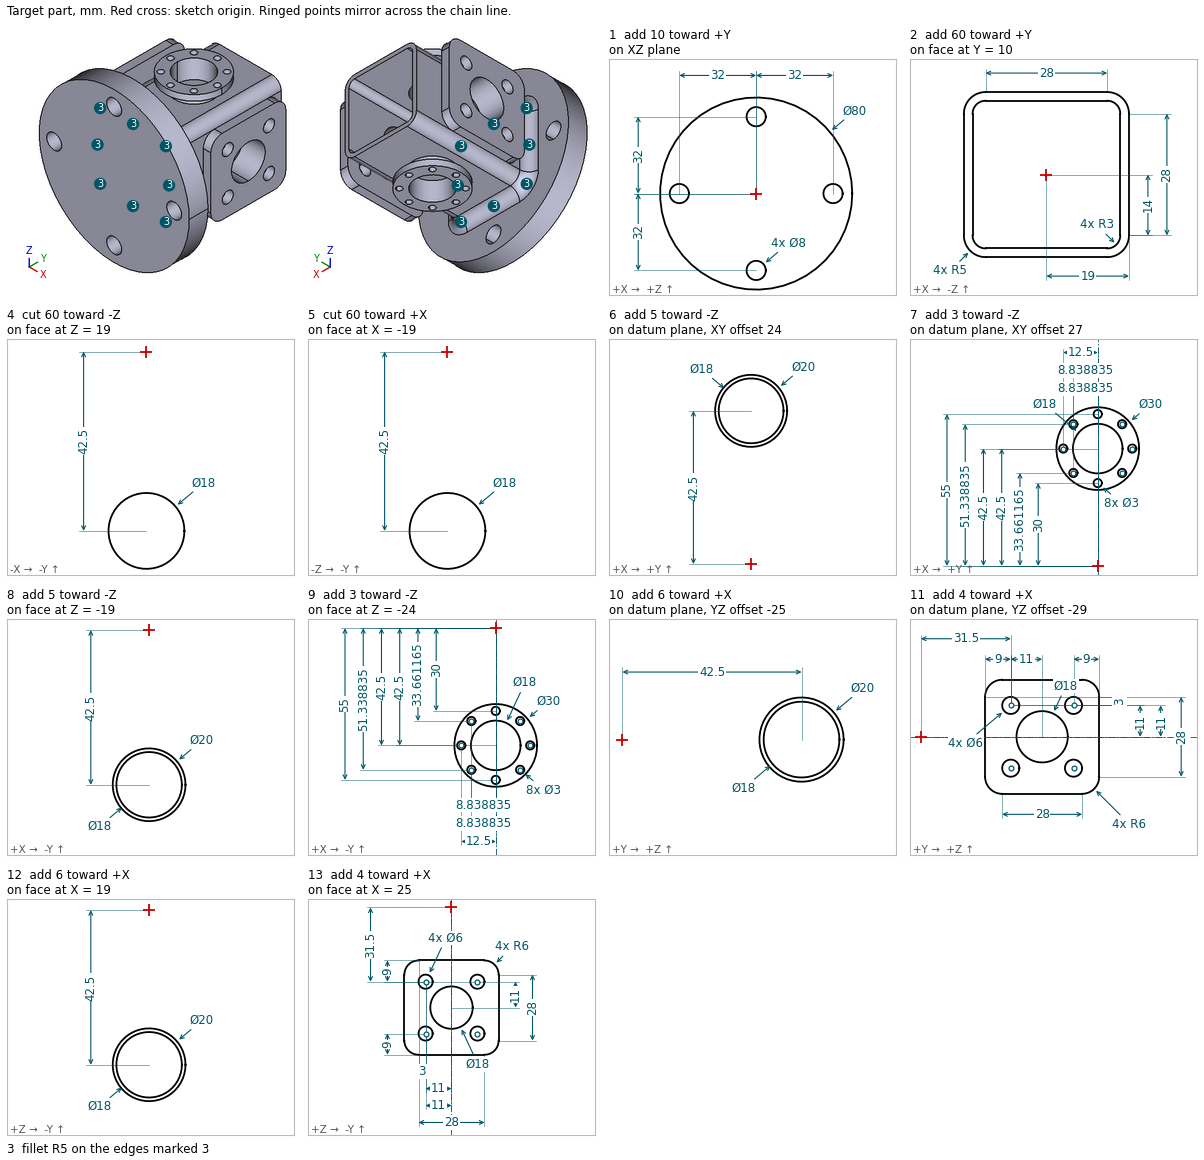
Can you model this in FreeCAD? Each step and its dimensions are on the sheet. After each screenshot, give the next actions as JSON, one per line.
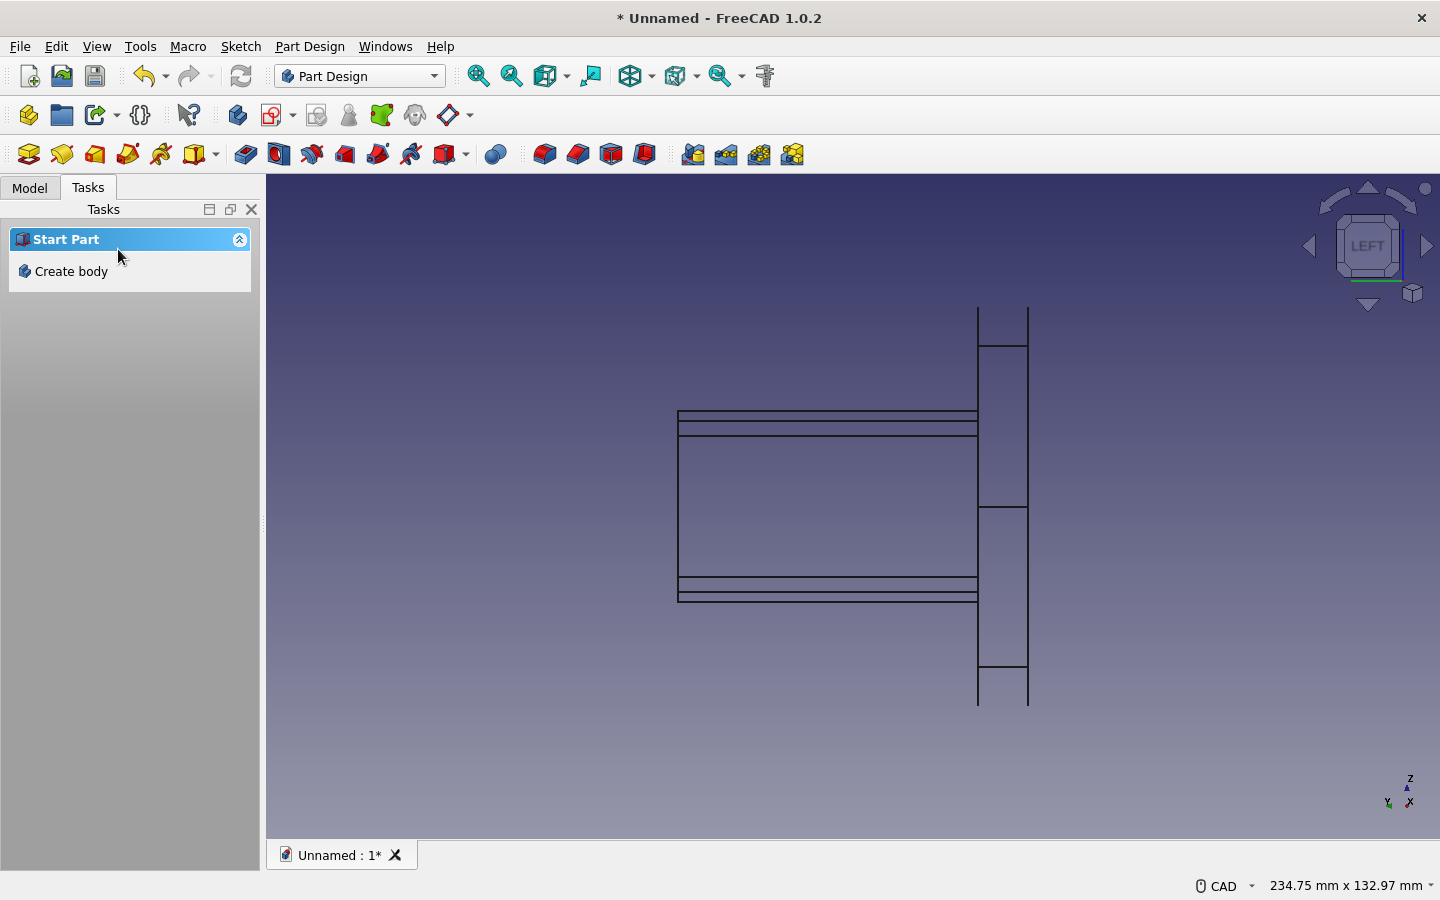
{"action": "key", "text": "0"}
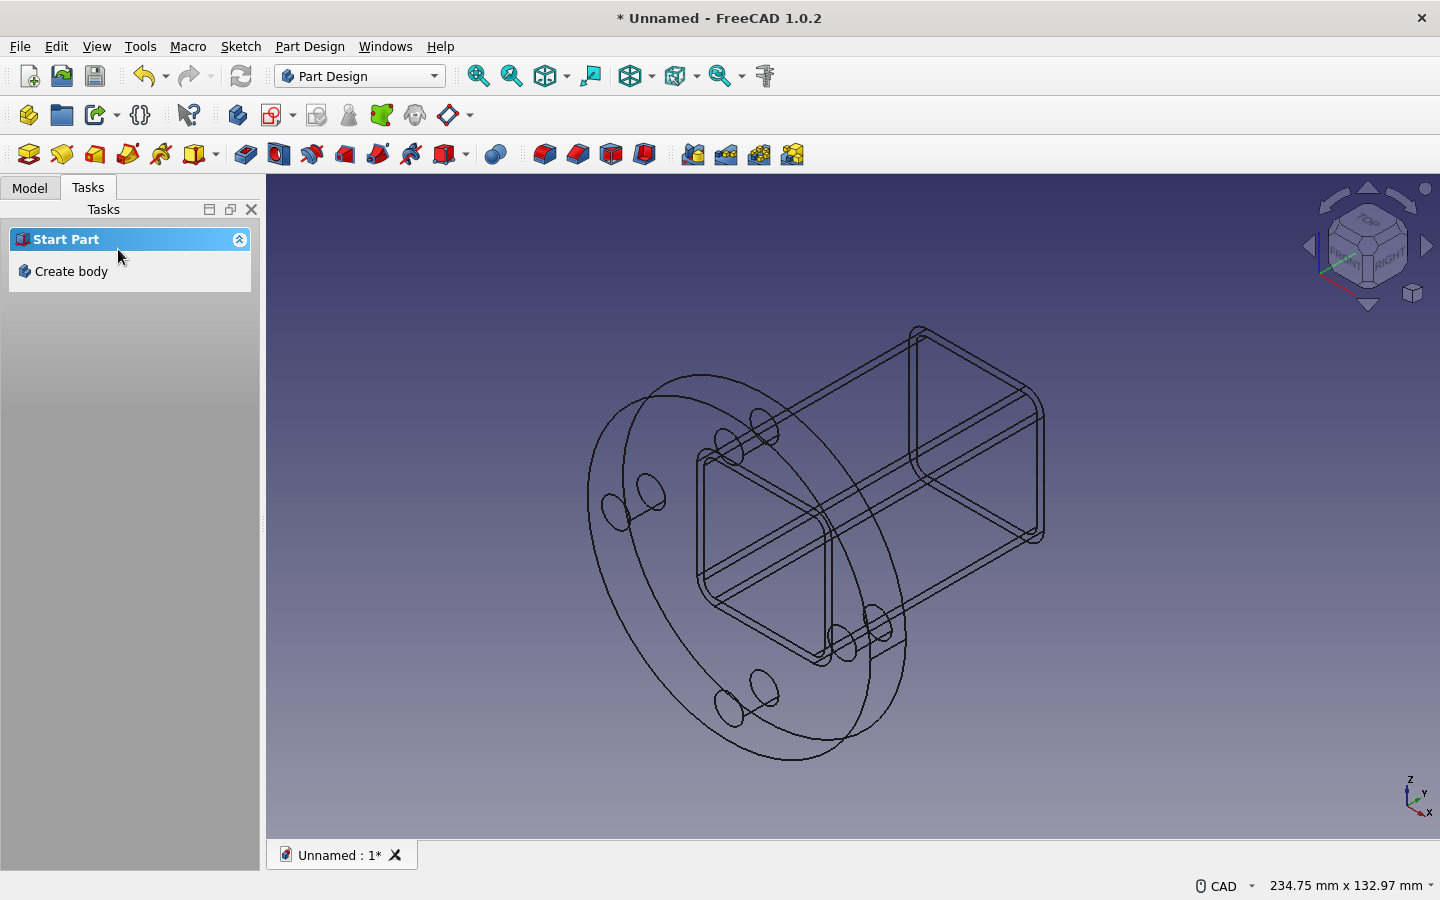
{"action": "left_click", "coordinate": [832, 595]}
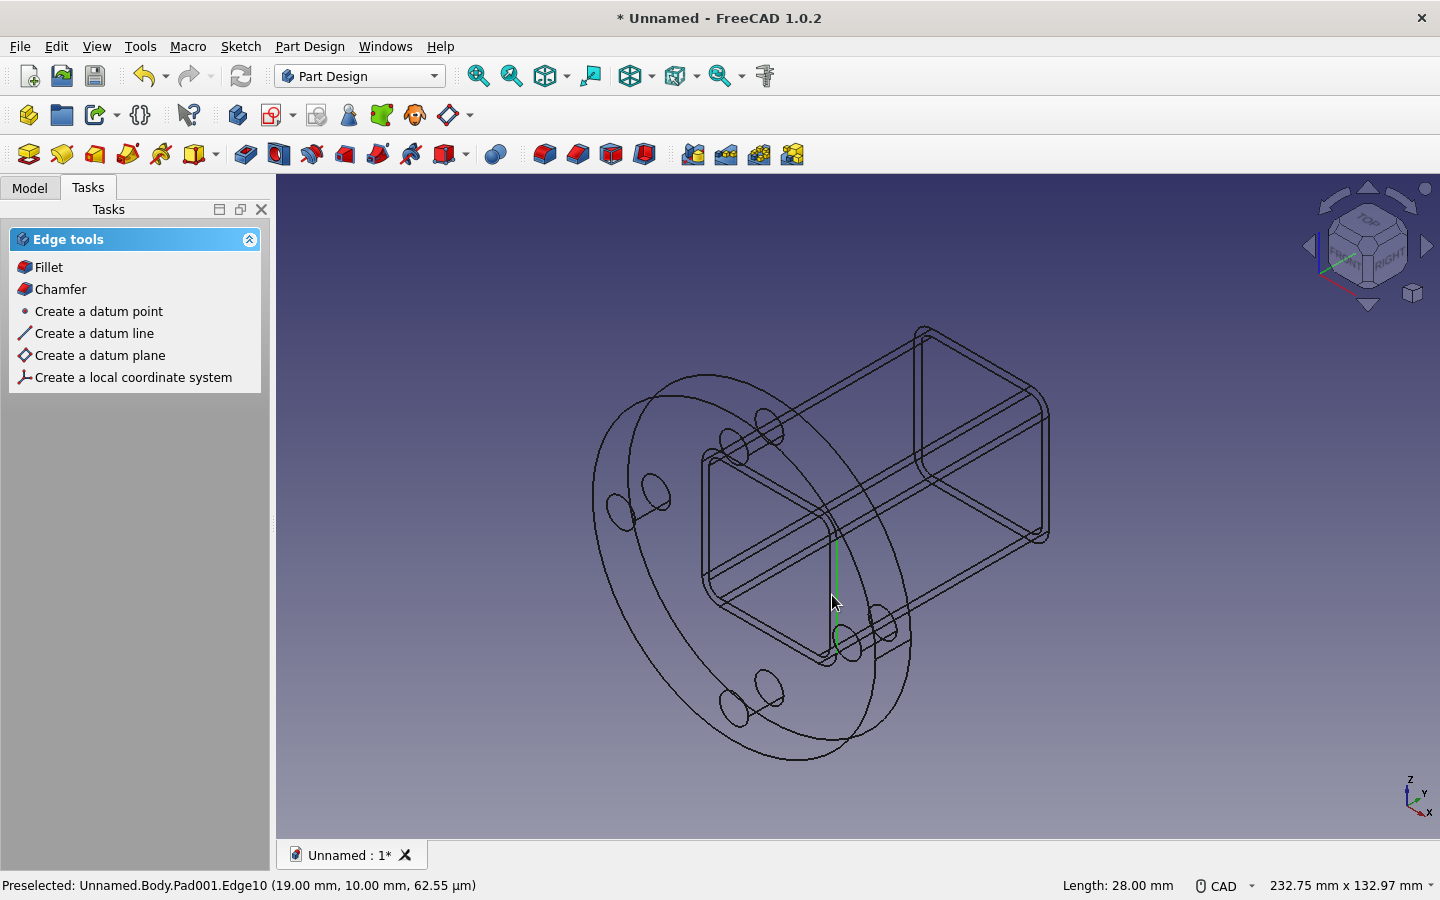
{"action": "left_click", "coordinate": [831, 664], "text": "ctrl"}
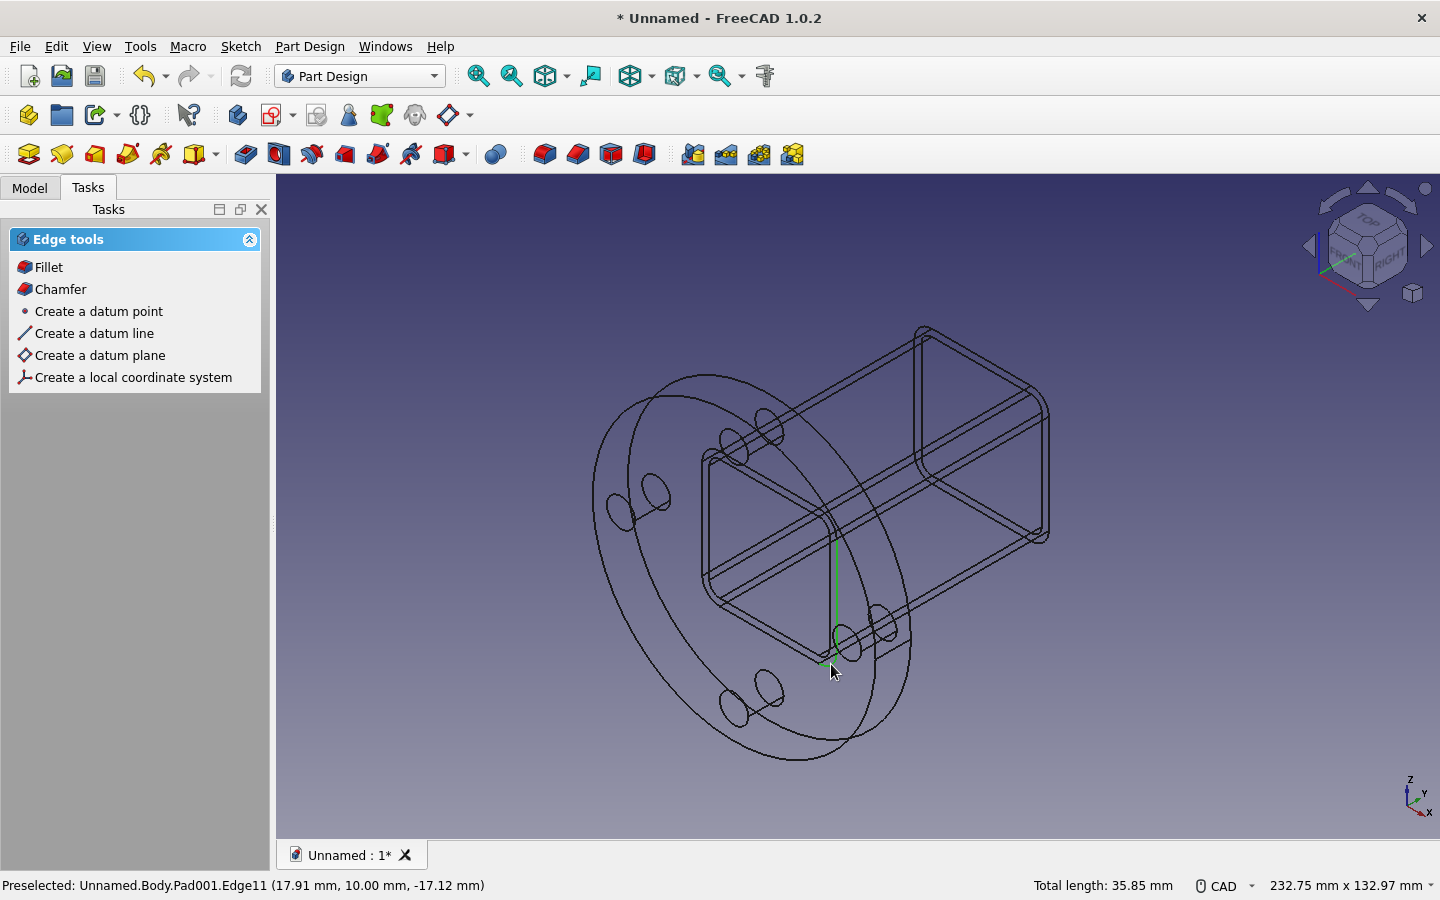
{"action": "left_click", "coordinate": [769, 634], "text": "ctrl"}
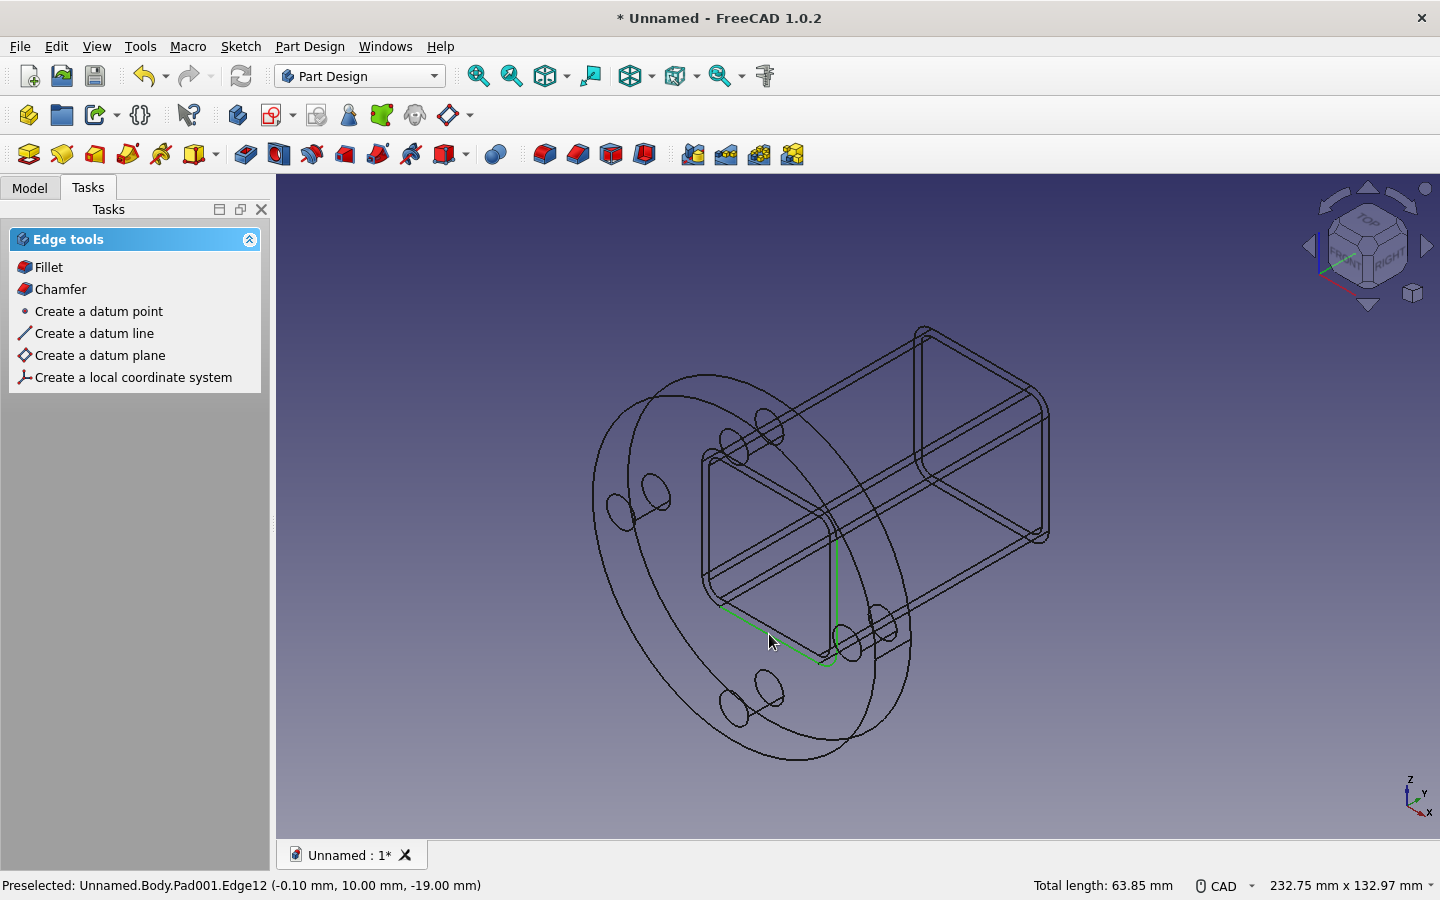
{"action": "left_click", "coordinate": [704, 585], "text": "ctrl"}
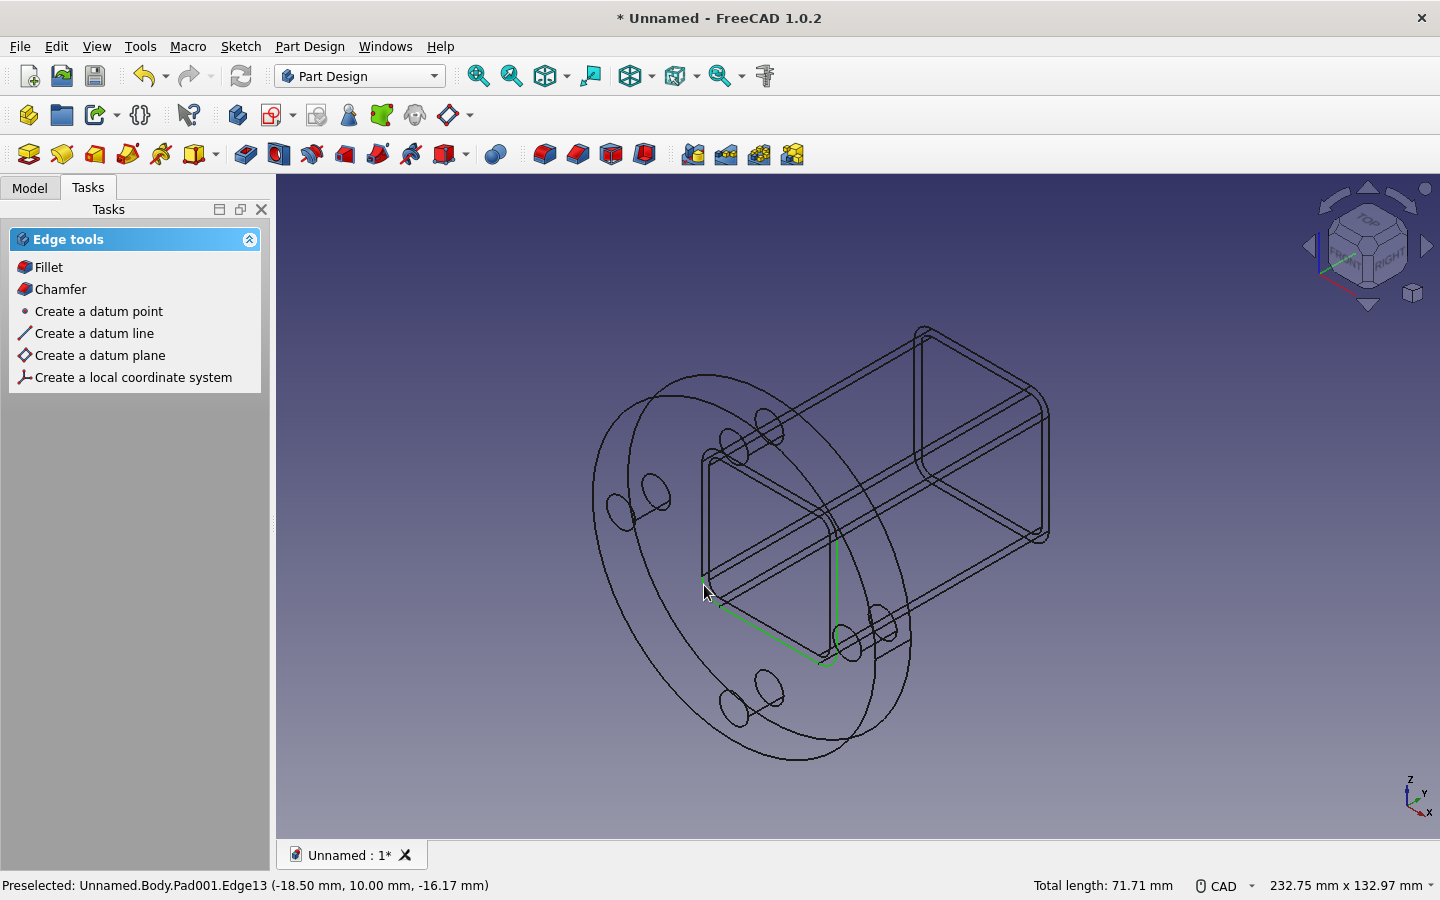
{"action": "left_click", "coordinate": [702, 518], "text": "ctrl"}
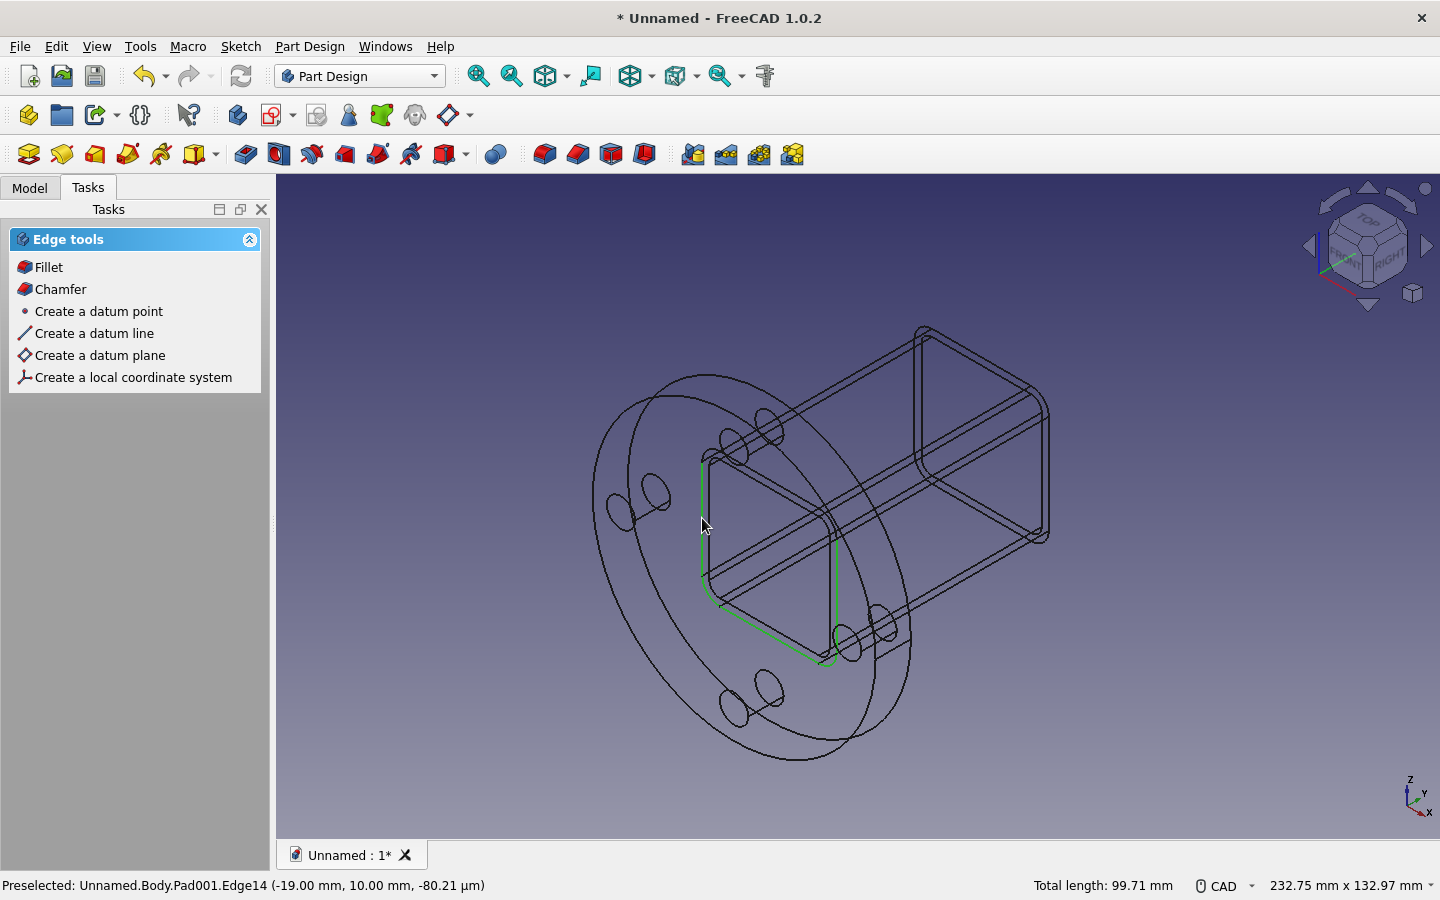
{"action": "left_click", "coordinate": [707, 449], "text": "ctrl"}